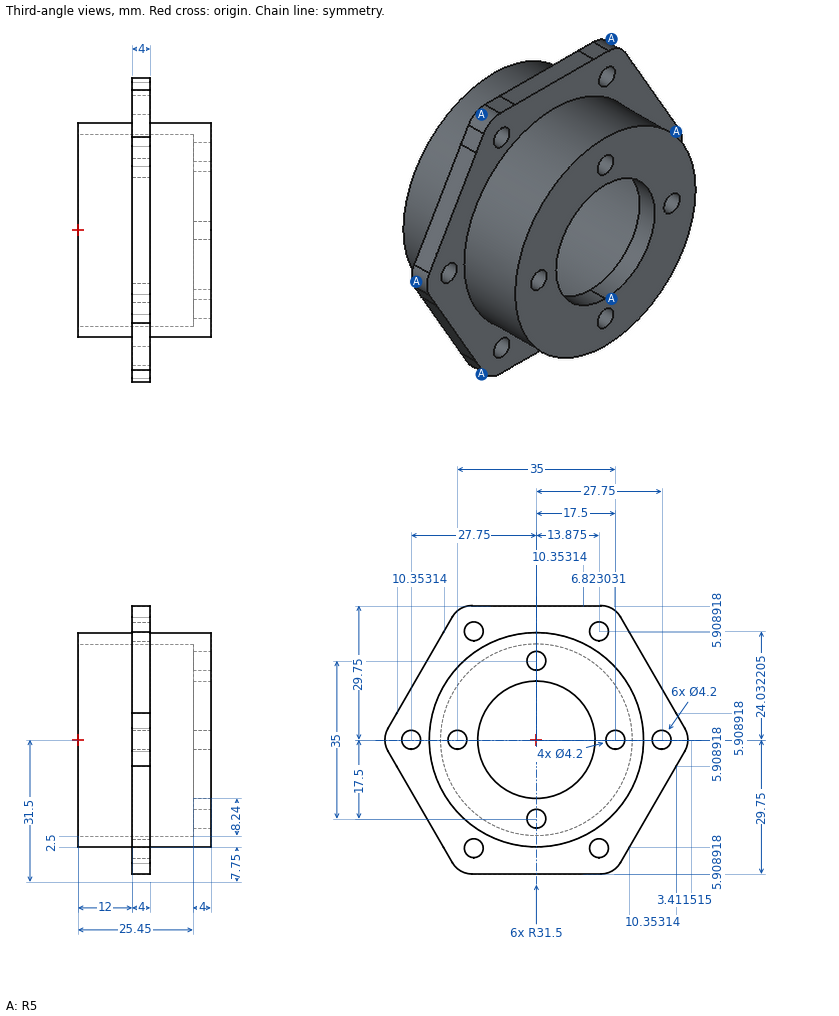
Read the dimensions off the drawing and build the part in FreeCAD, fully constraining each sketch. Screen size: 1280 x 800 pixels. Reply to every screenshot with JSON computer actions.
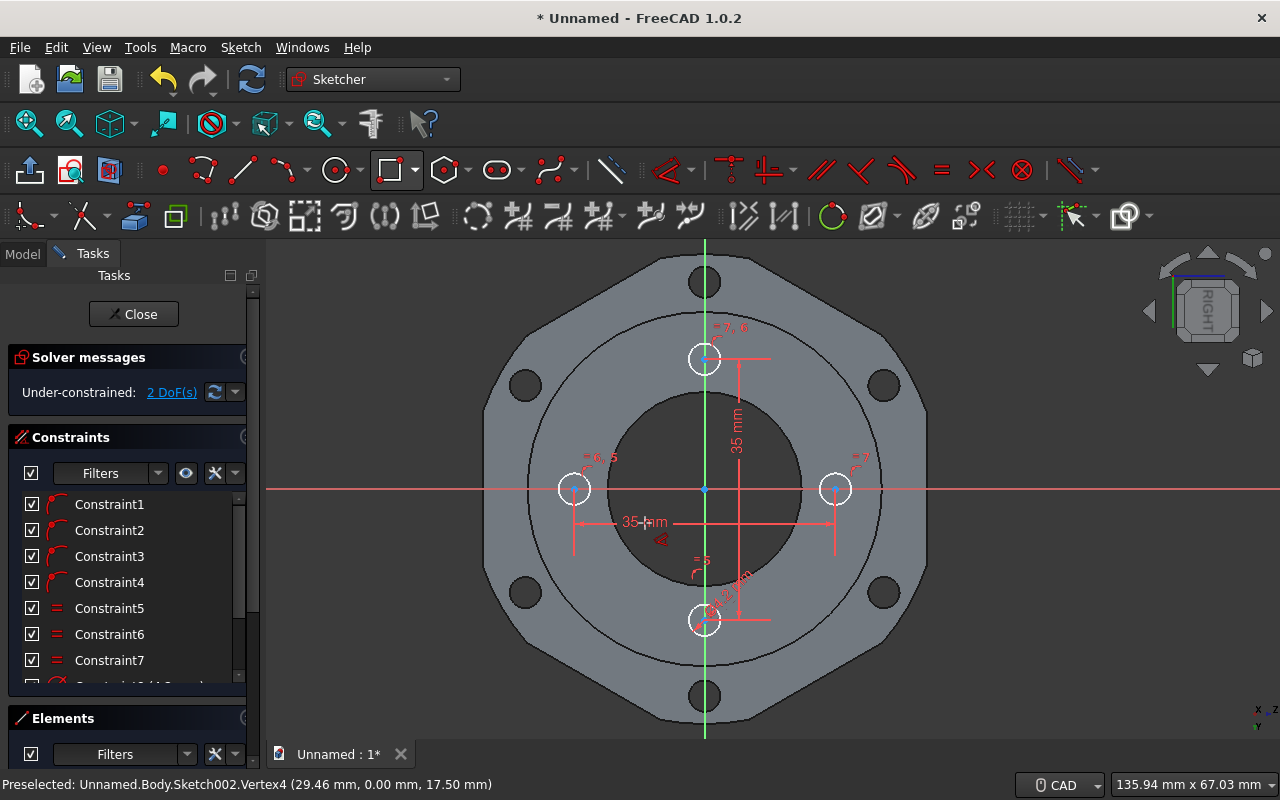
{"action": "left_click", "coordinate": [705, 620]}
{"action": "left_click", "coordinate": [739, 555]}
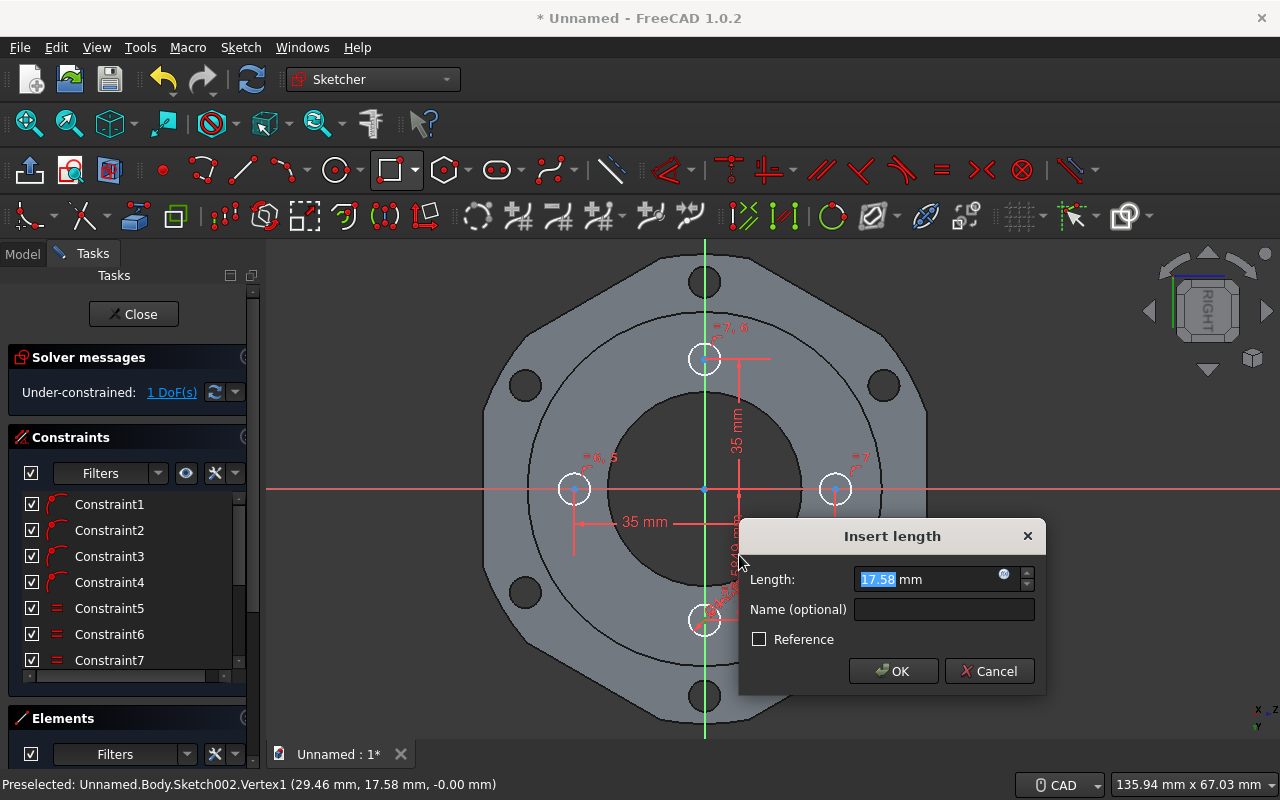
{"action": "type", "text": "17.5"}
{"action": "key", "text": "Return"}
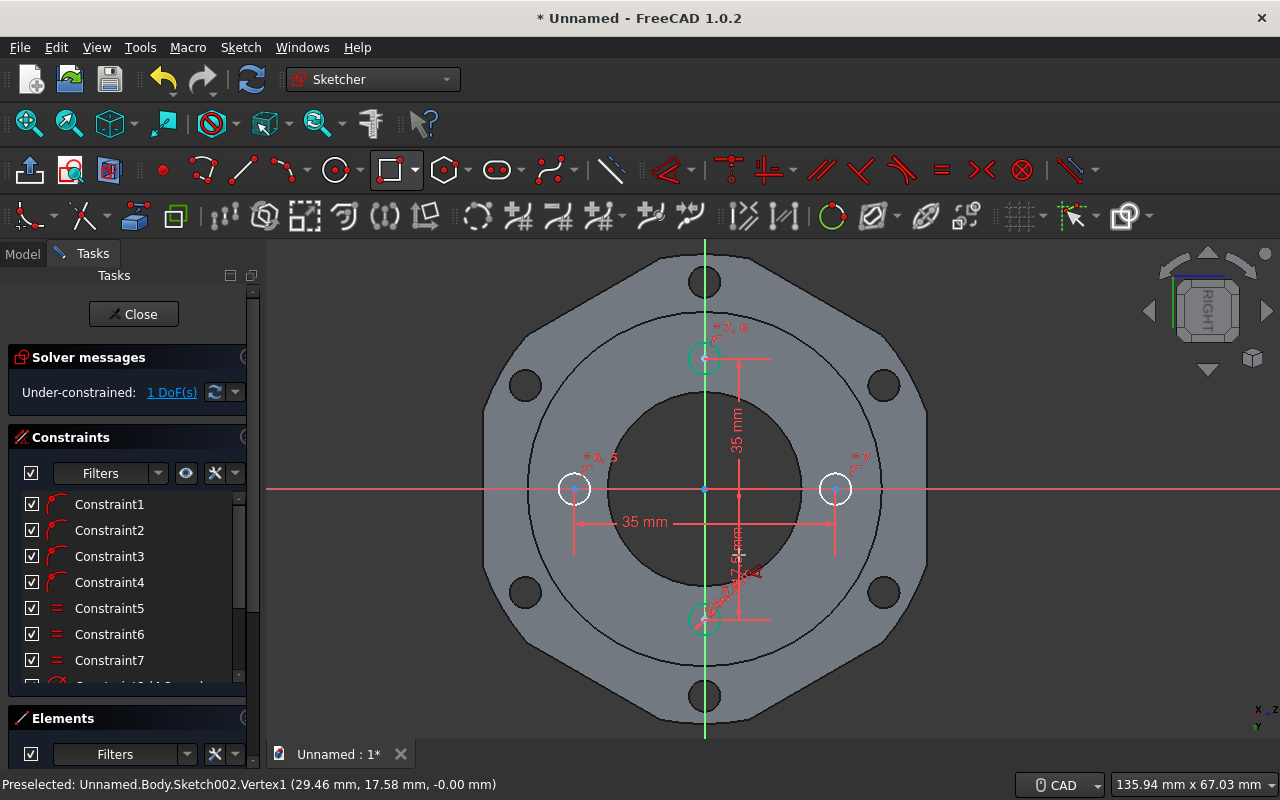
{"action": "left_click", "coordinate": [574, 489]}
{"action": "left_click", "coordinate": [640, 455]}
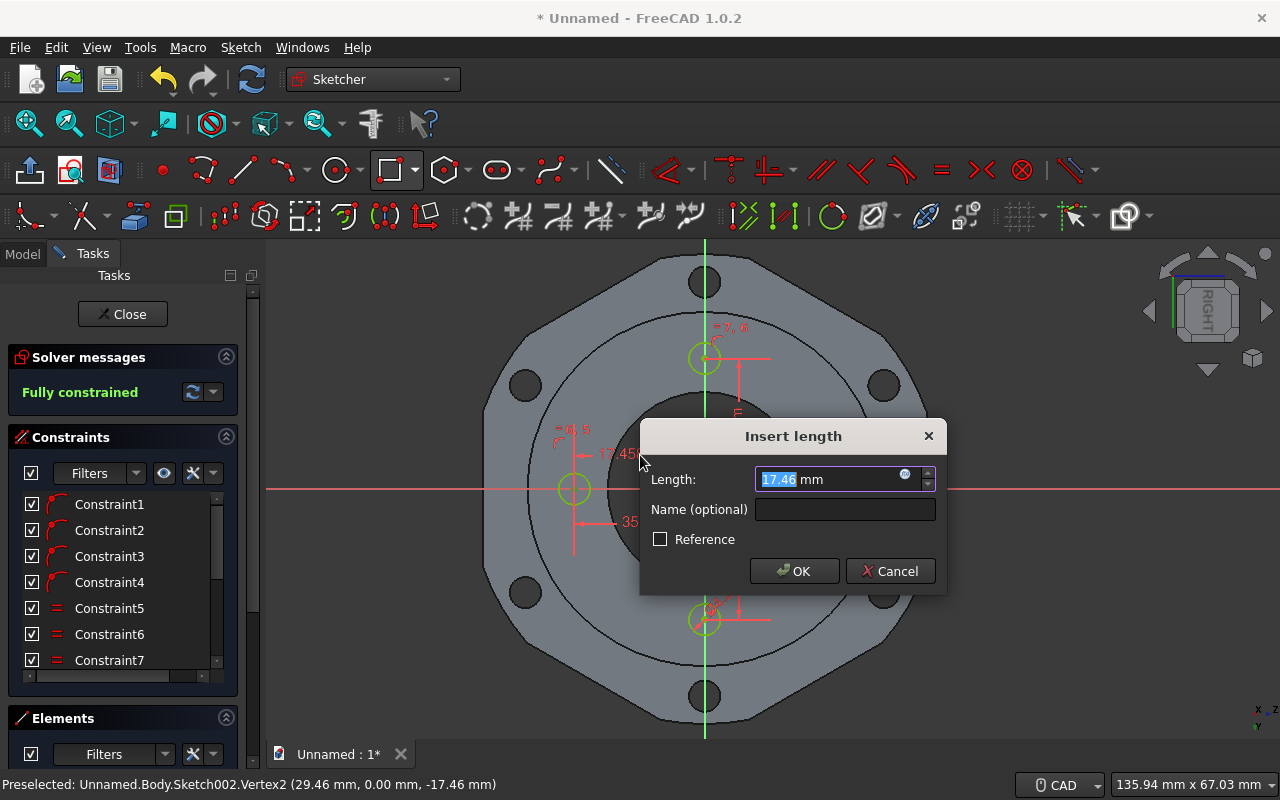
{"action": "type", "text": "17.5"}
{"action": "key", "text": "Return"}
{"action": "key", "text": "Escape"}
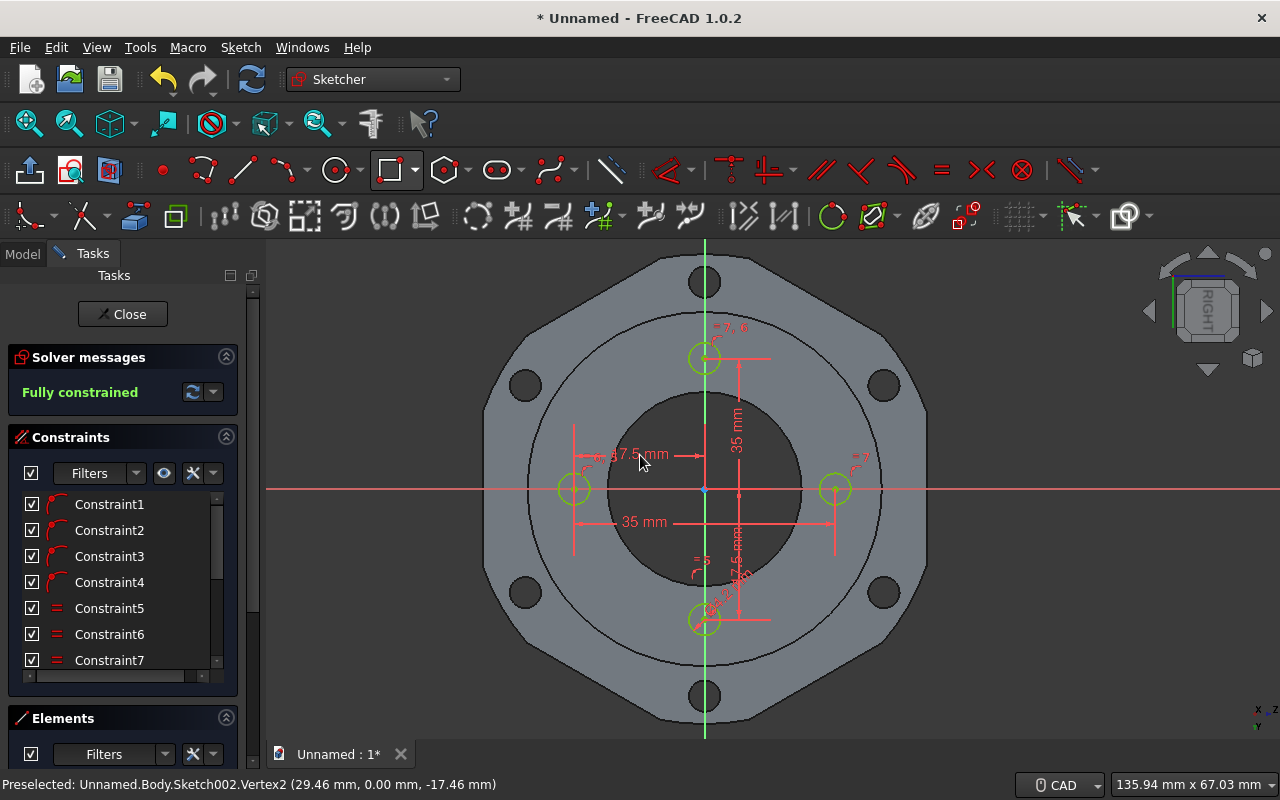
{"action": "left_click", "coordinate": [123, 314]}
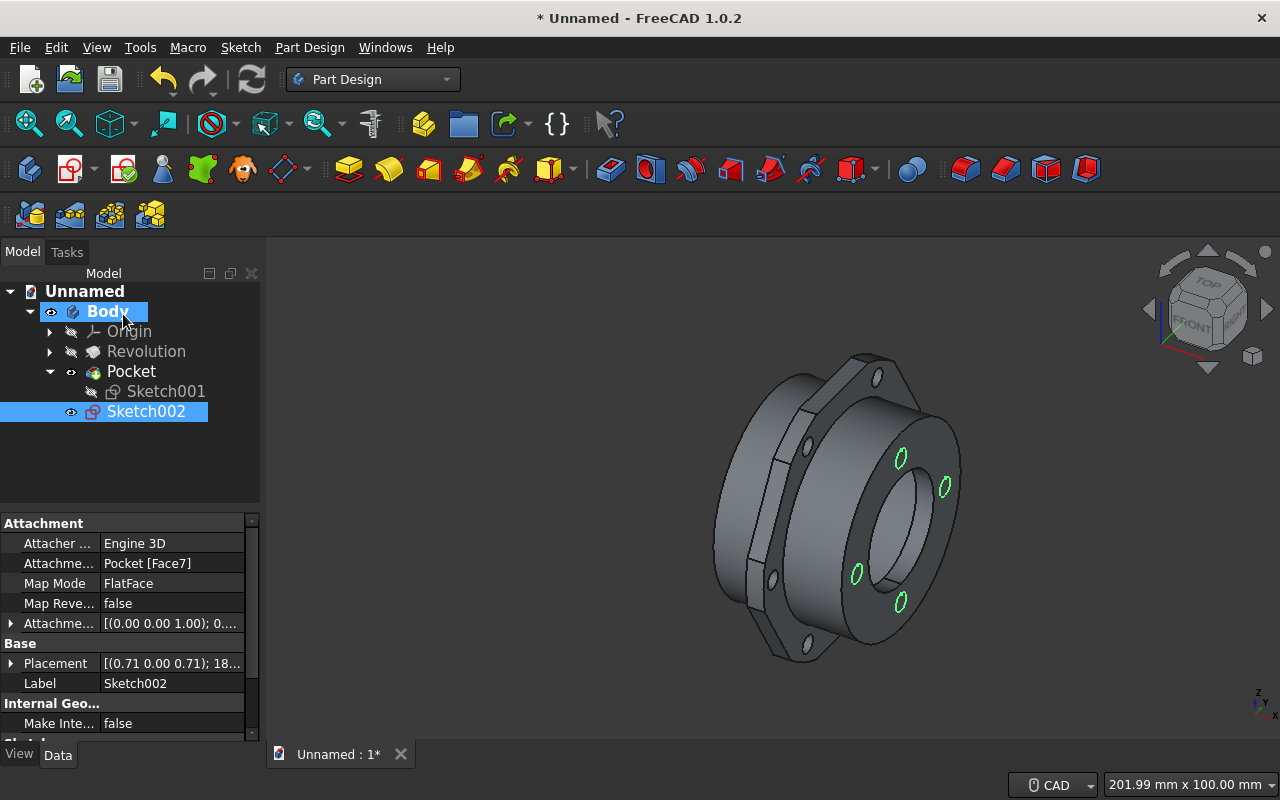
{"action": "left_click", "coordinate": [612, 170]}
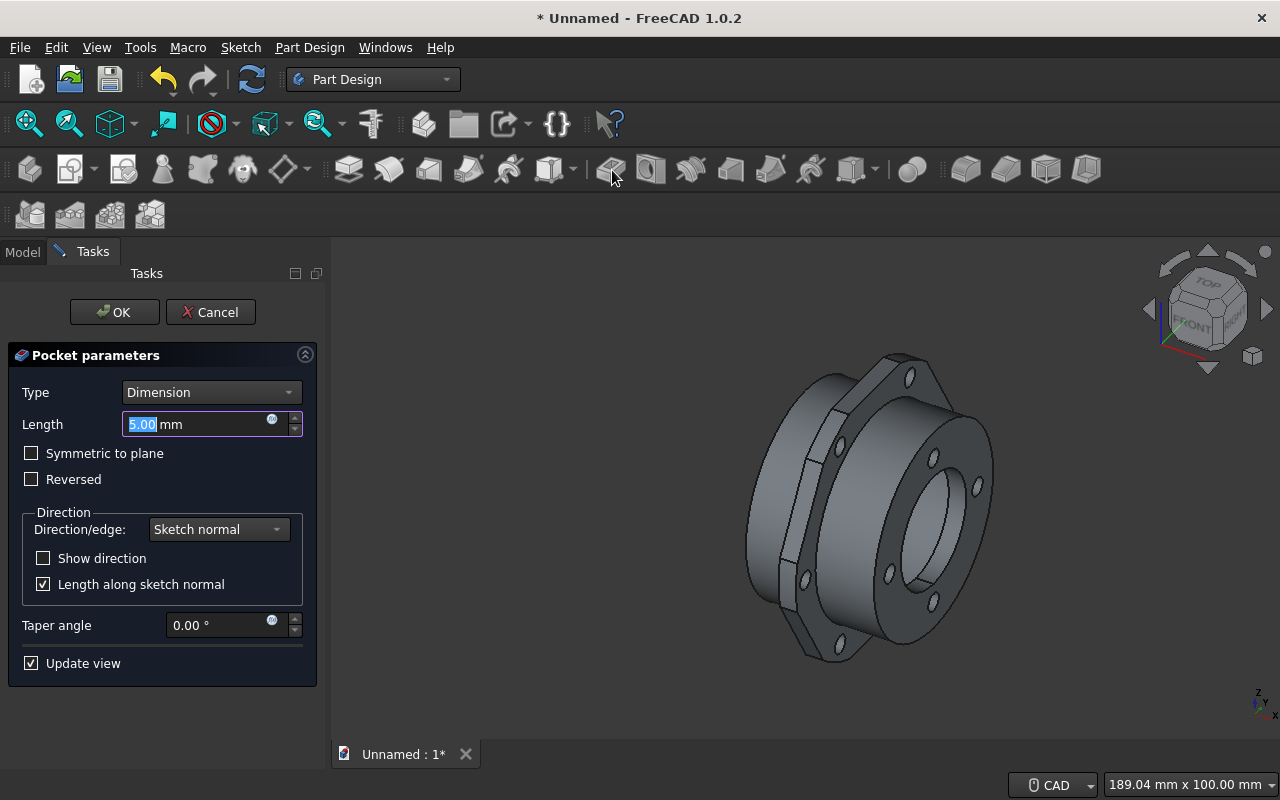
{"action": "left_click", "coordinate": [212, 392]}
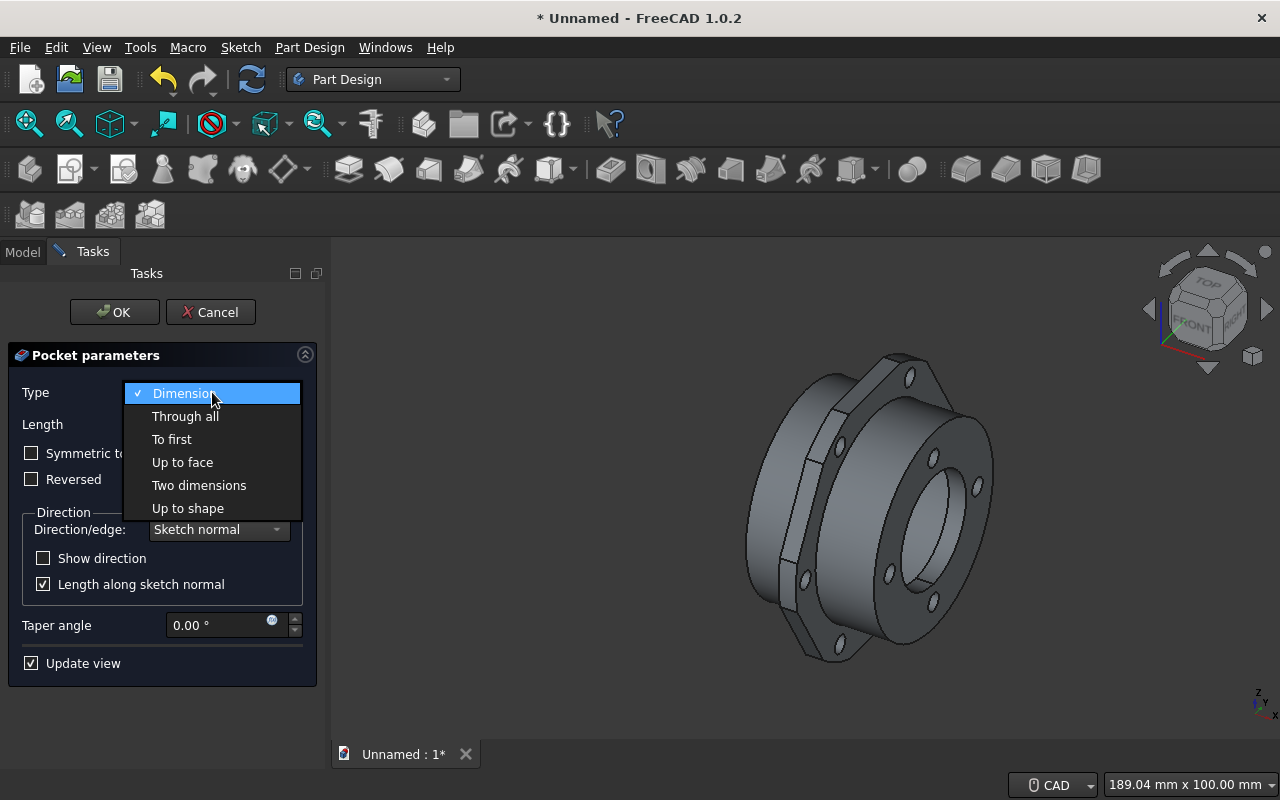
{"action": "left_click", "coordinate": [212, 416]}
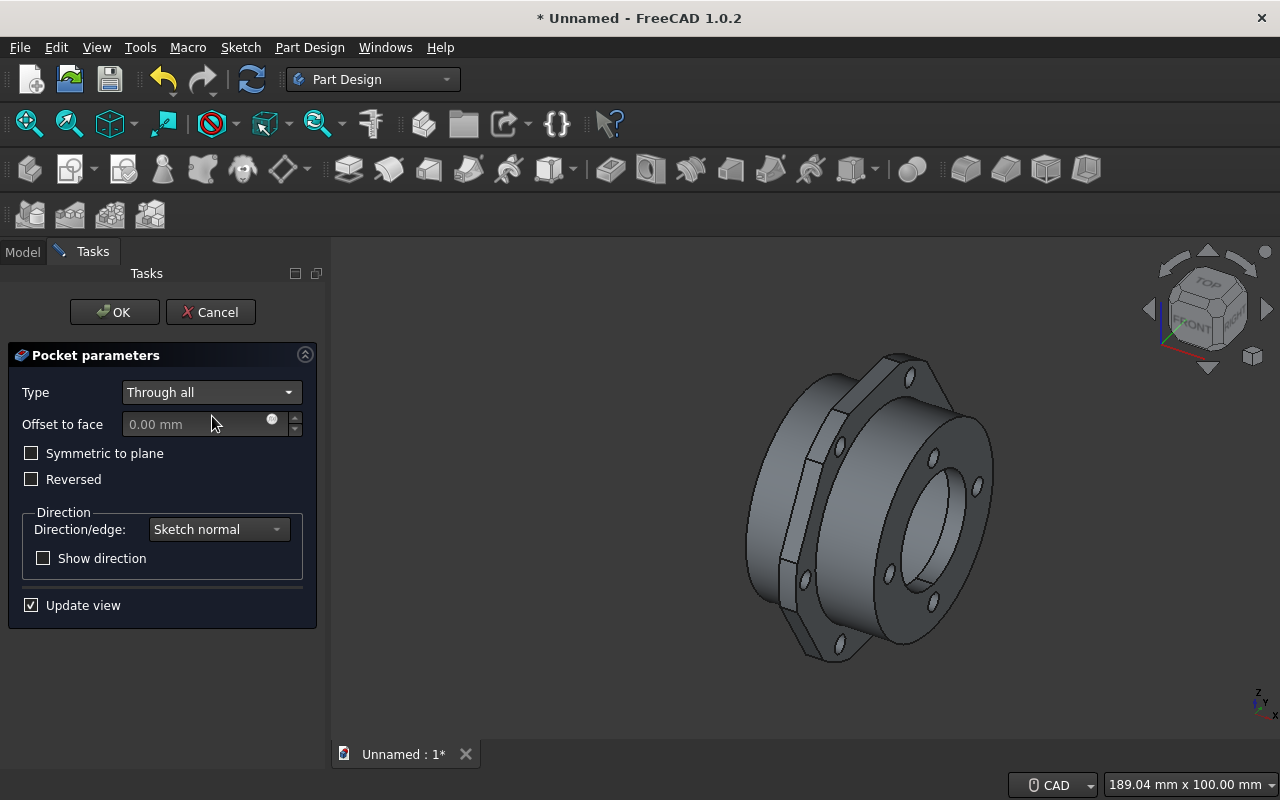
{"action": "left_click", "coordinate": [115, 312]}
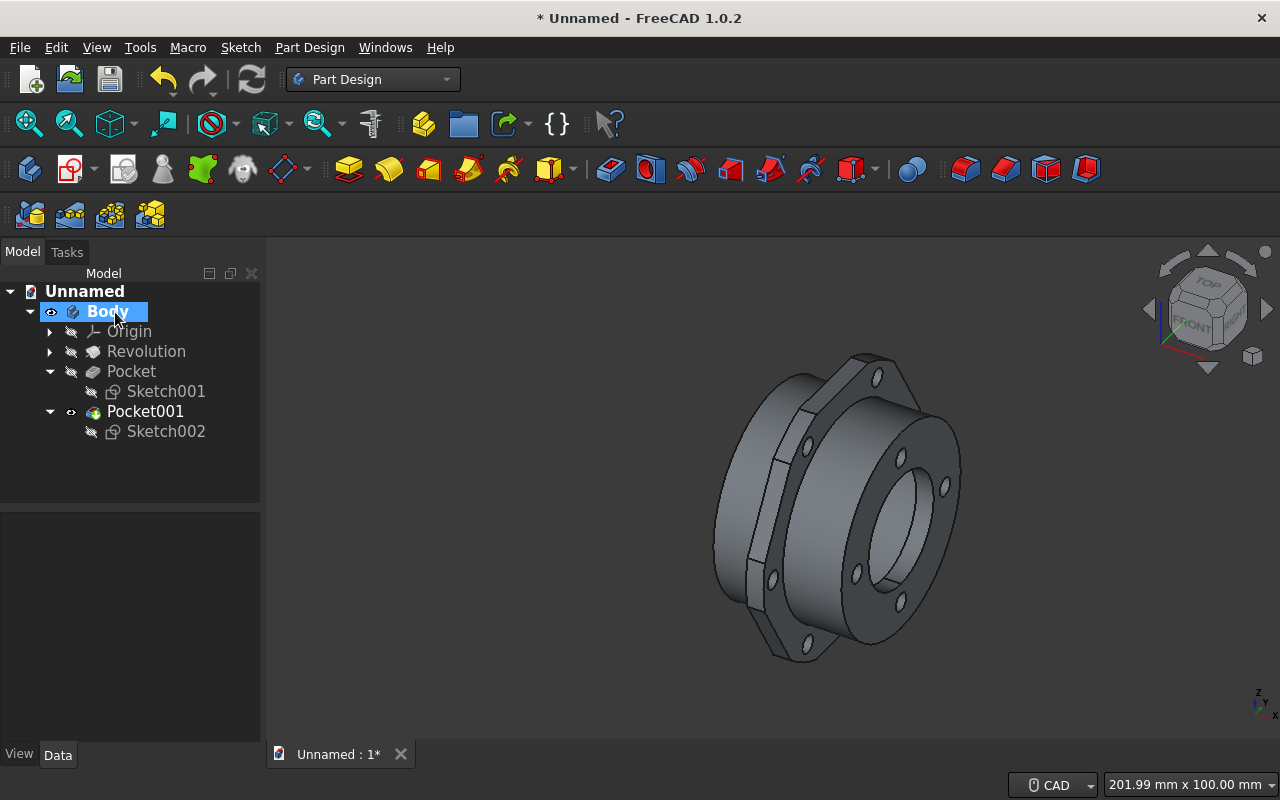
{"action": "left_click", "coordinate": [820, 428]}